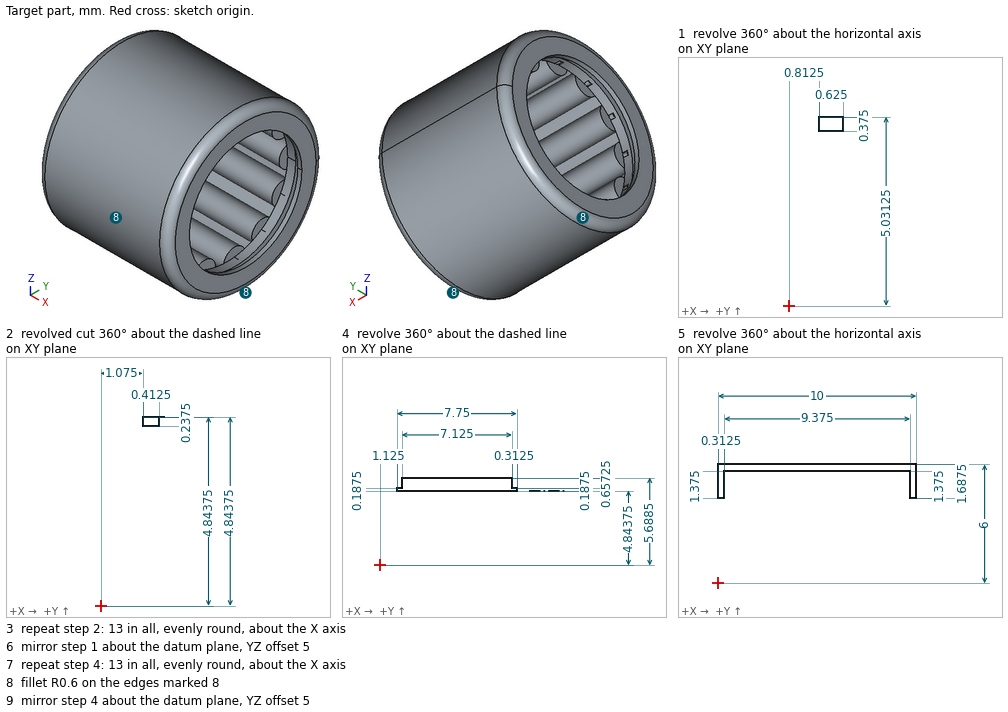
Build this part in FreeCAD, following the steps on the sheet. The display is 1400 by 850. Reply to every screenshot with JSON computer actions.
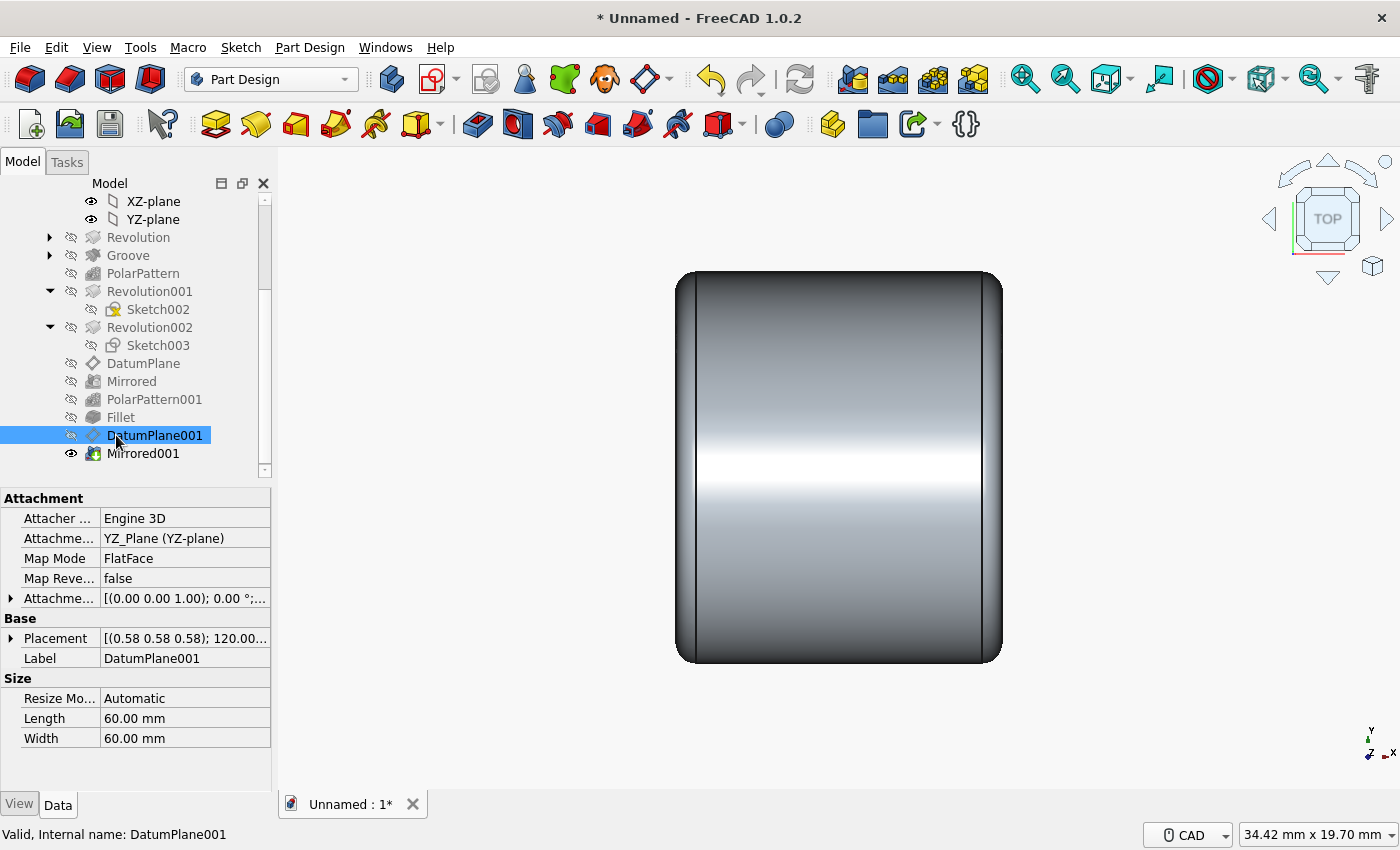
{"action": "key", "text": "0"}